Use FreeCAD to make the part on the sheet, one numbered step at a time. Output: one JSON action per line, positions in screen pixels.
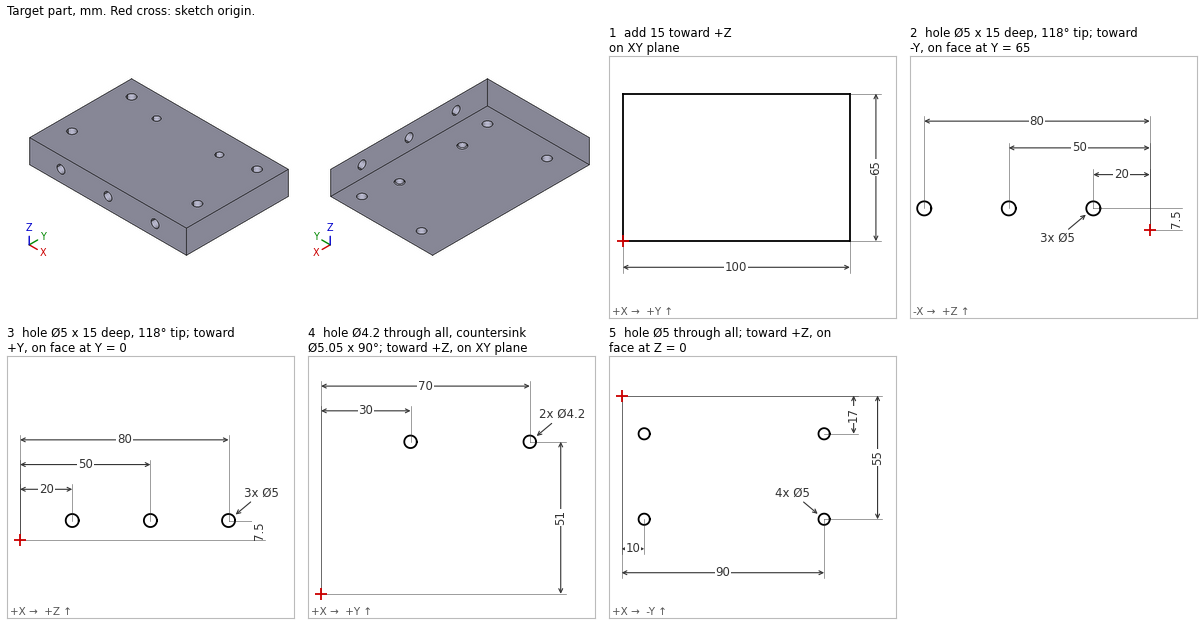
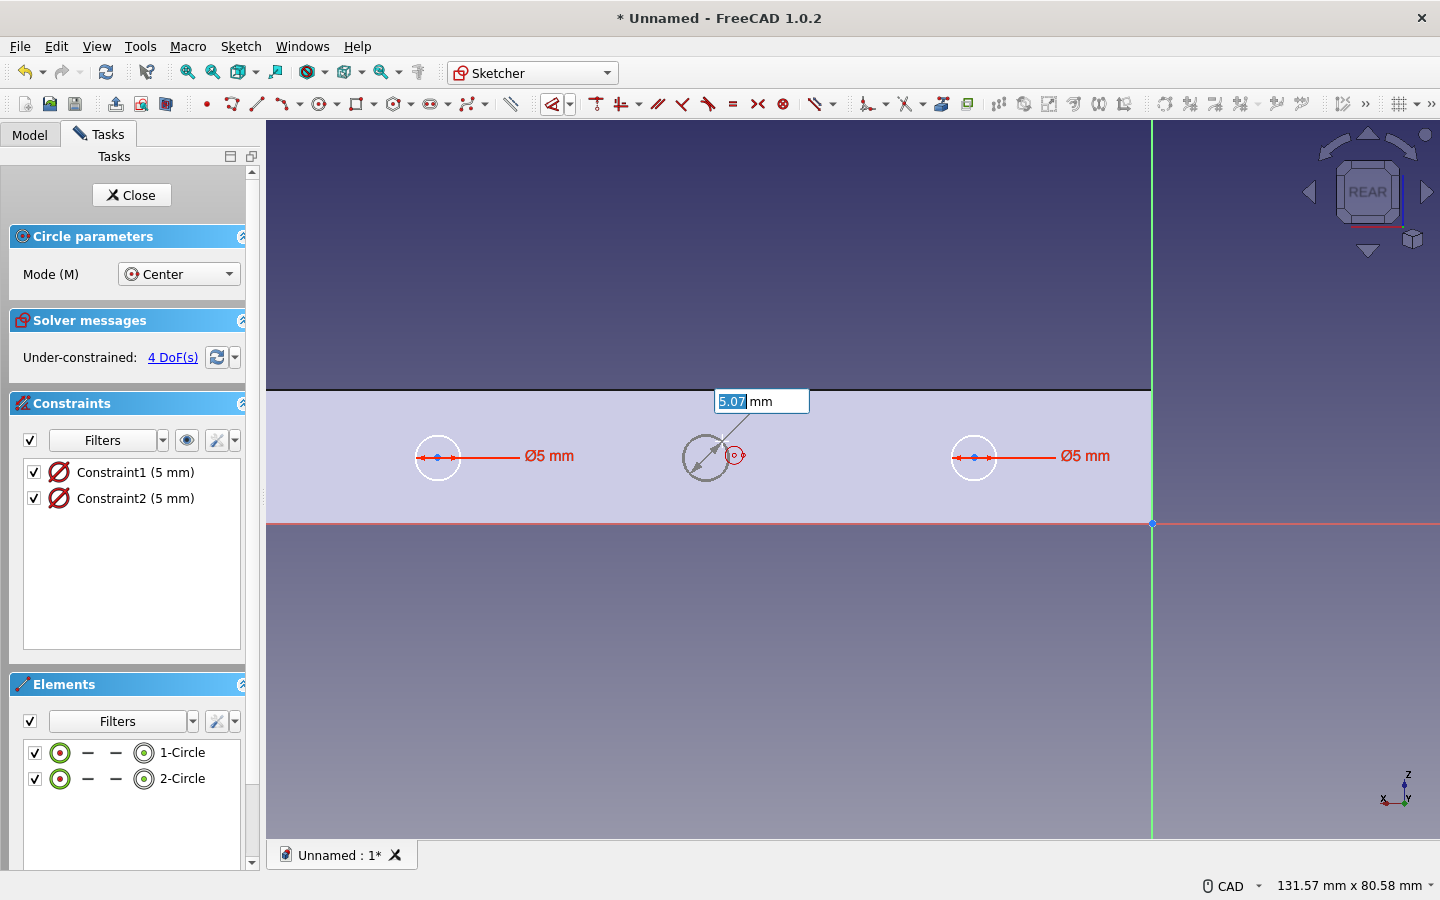
{"action": "type", "text": "5"}
{"action": "key", "text": "Return"}
{"action": "key", "text": "Escape"}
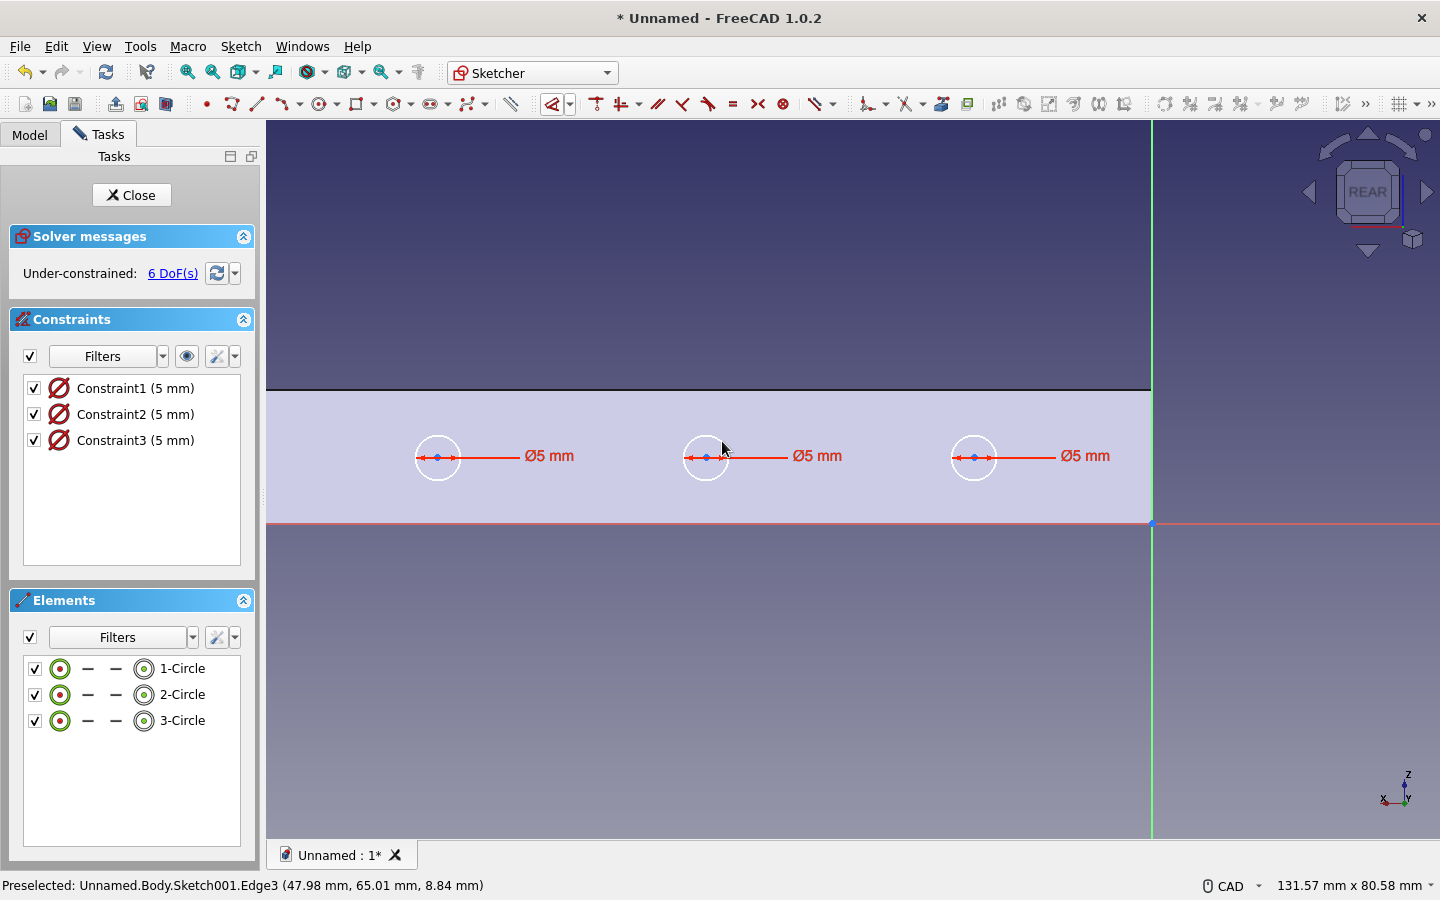
{"action": "left_click", "coordinate": [974, 458]}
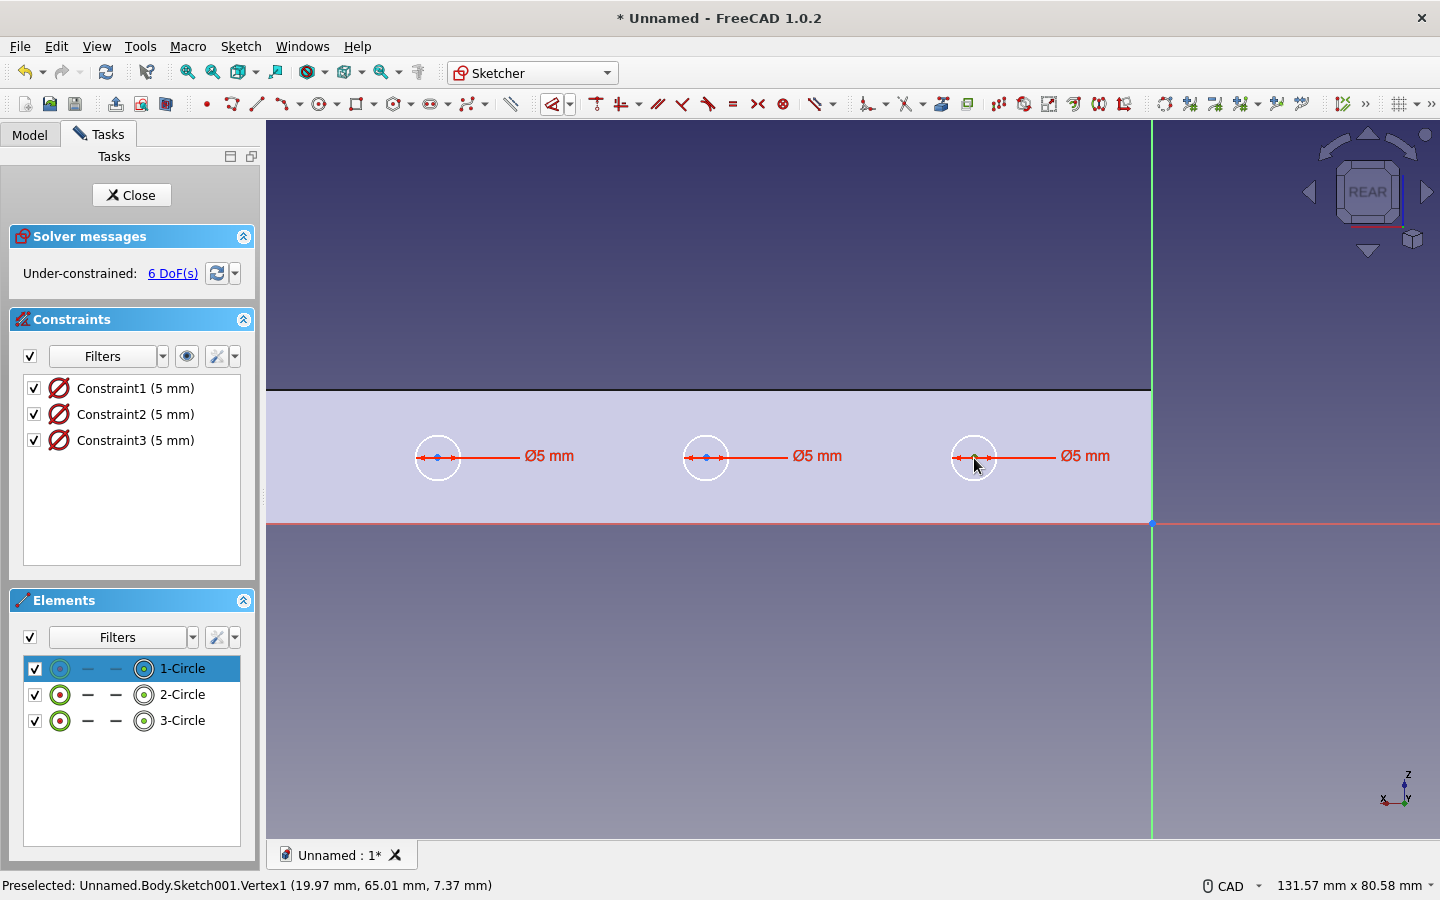
{"action": "left_click", "coordinate": [438, 458]}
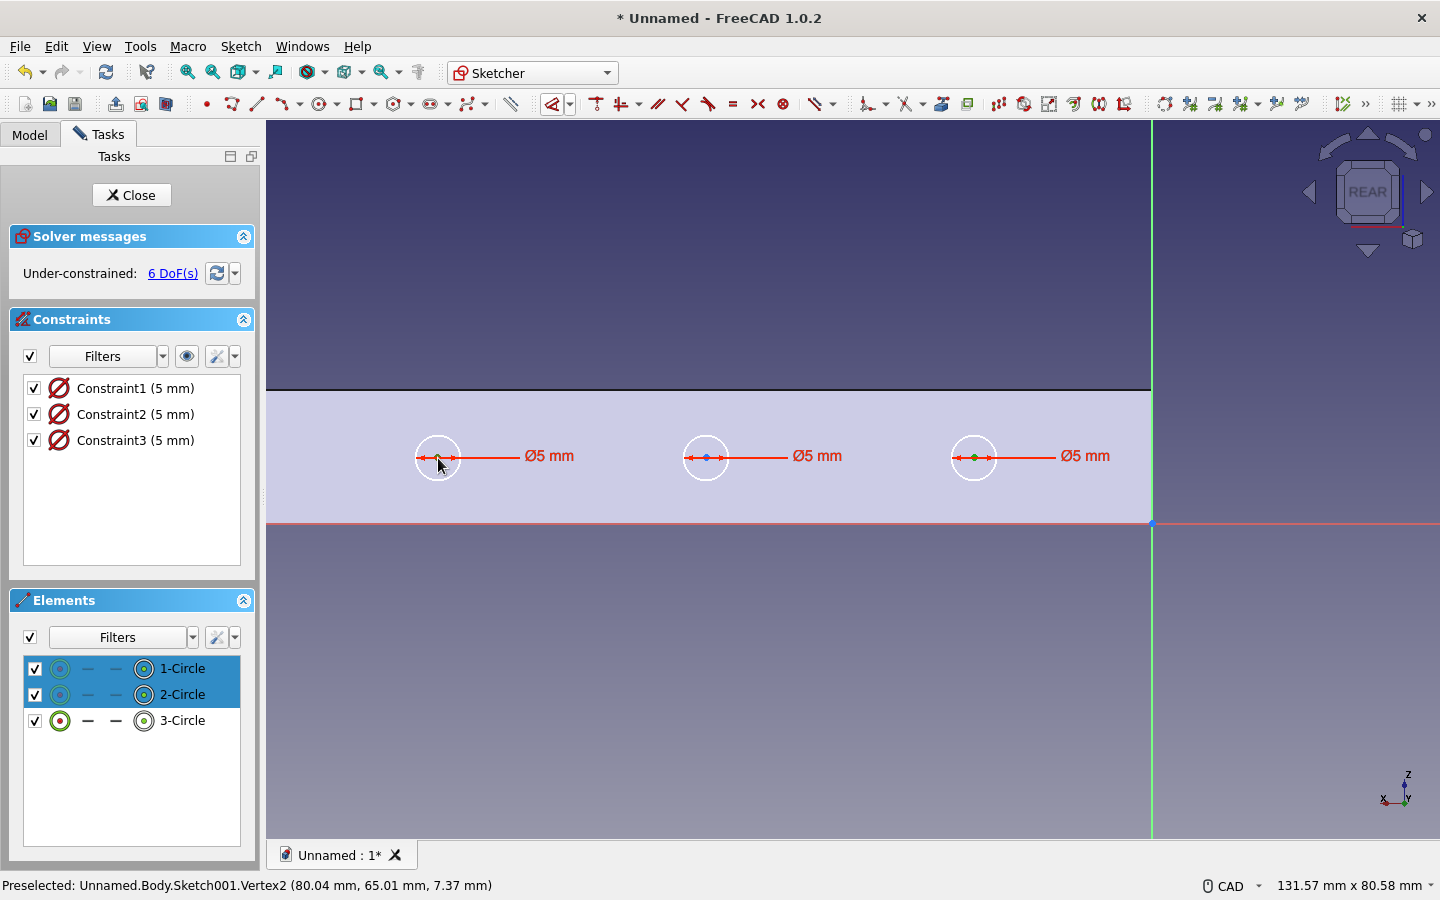
{"action": "key", "text": "h"}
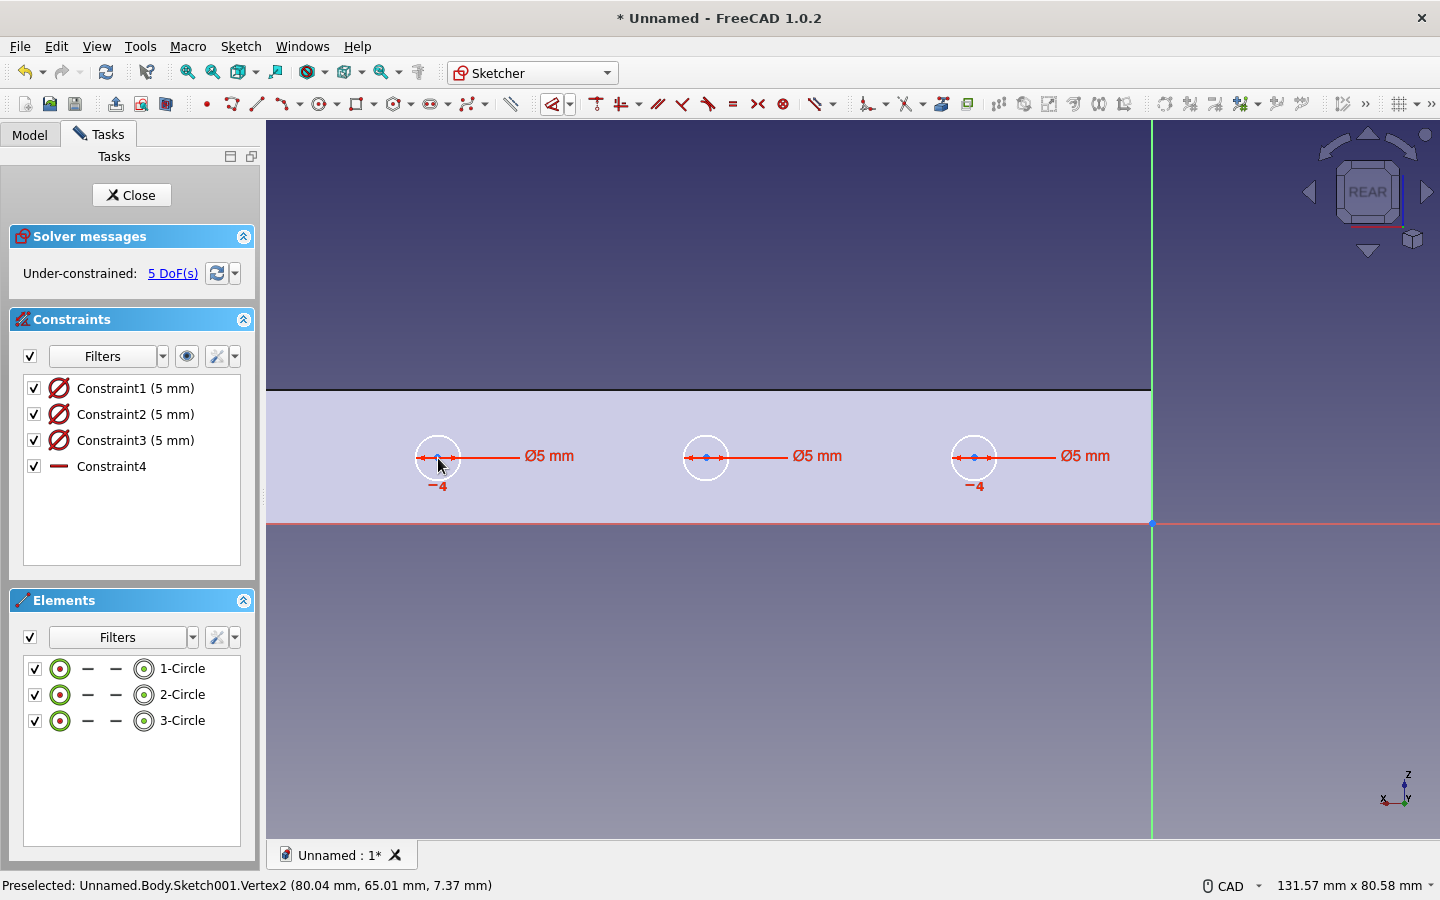
{"action": "left_click", "coordinate": [974, 458]}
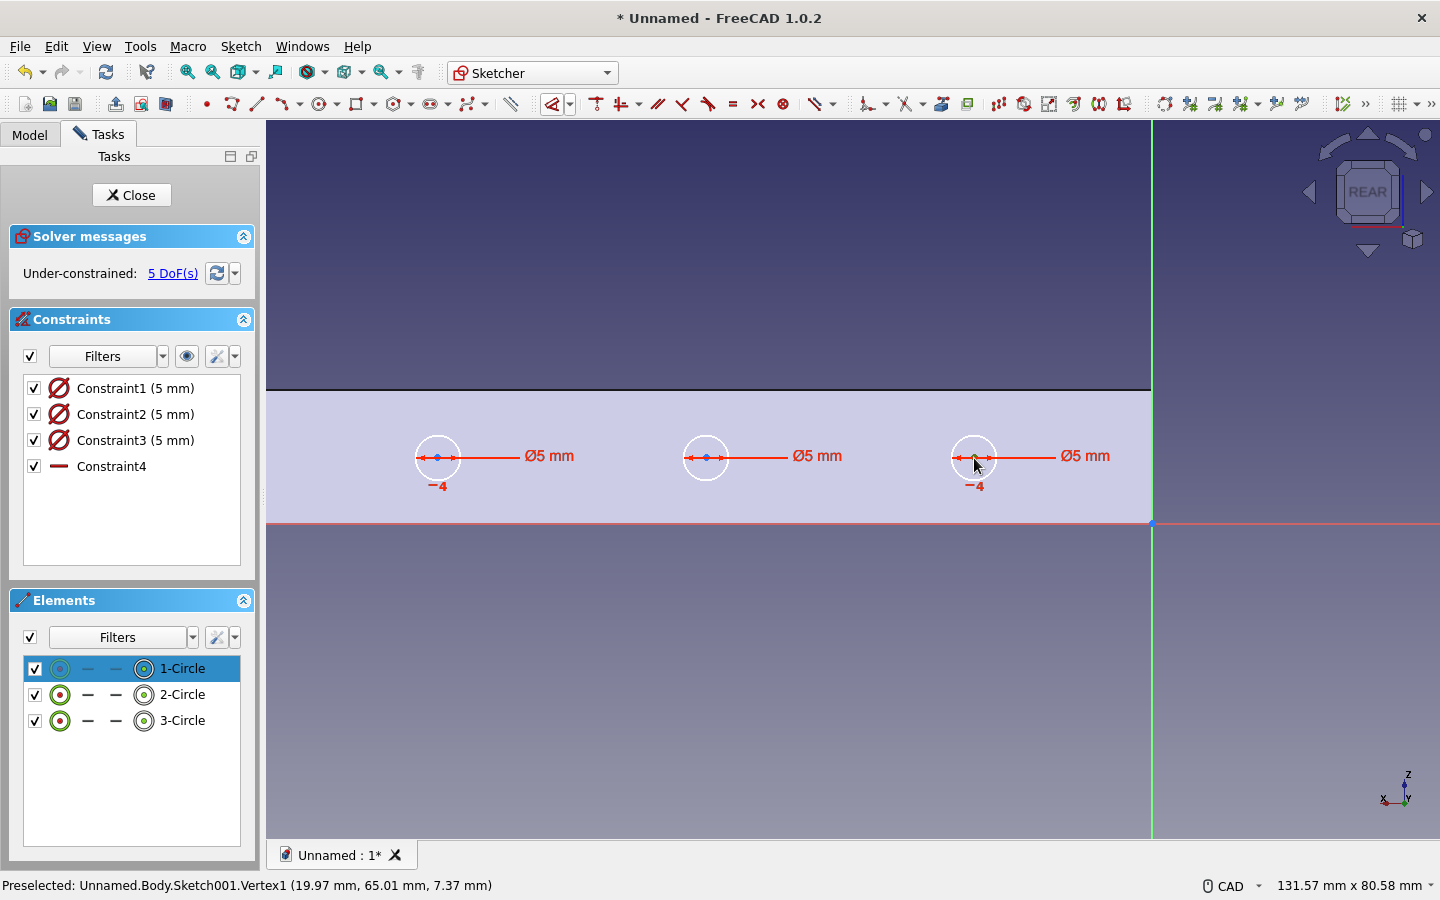
{"action": "left_click", "coordinate": [706, 458]}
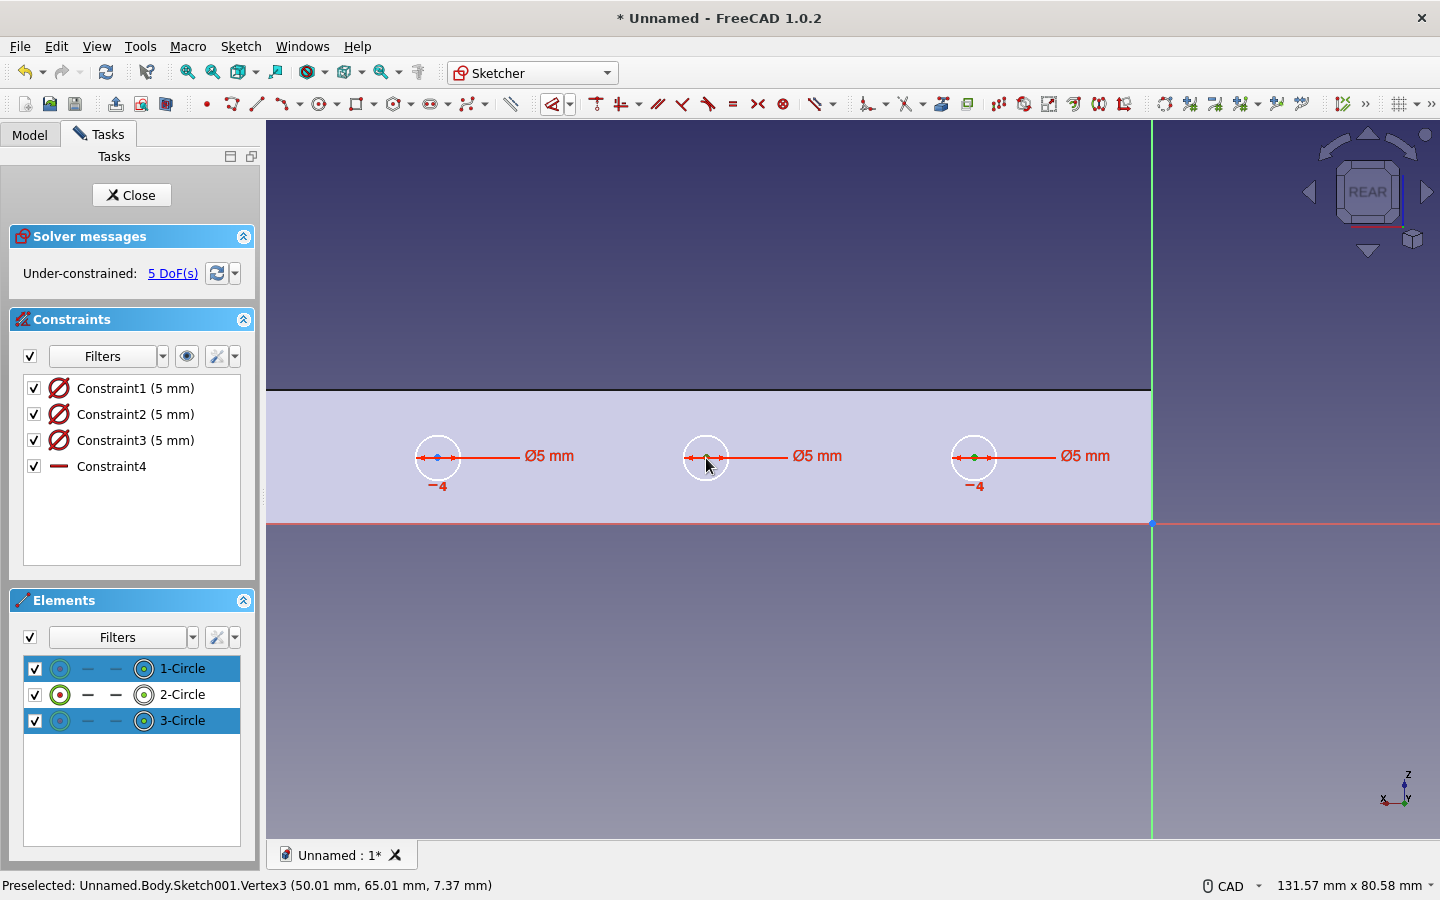
{"action": "left_click", "coordinate": [638, 104]}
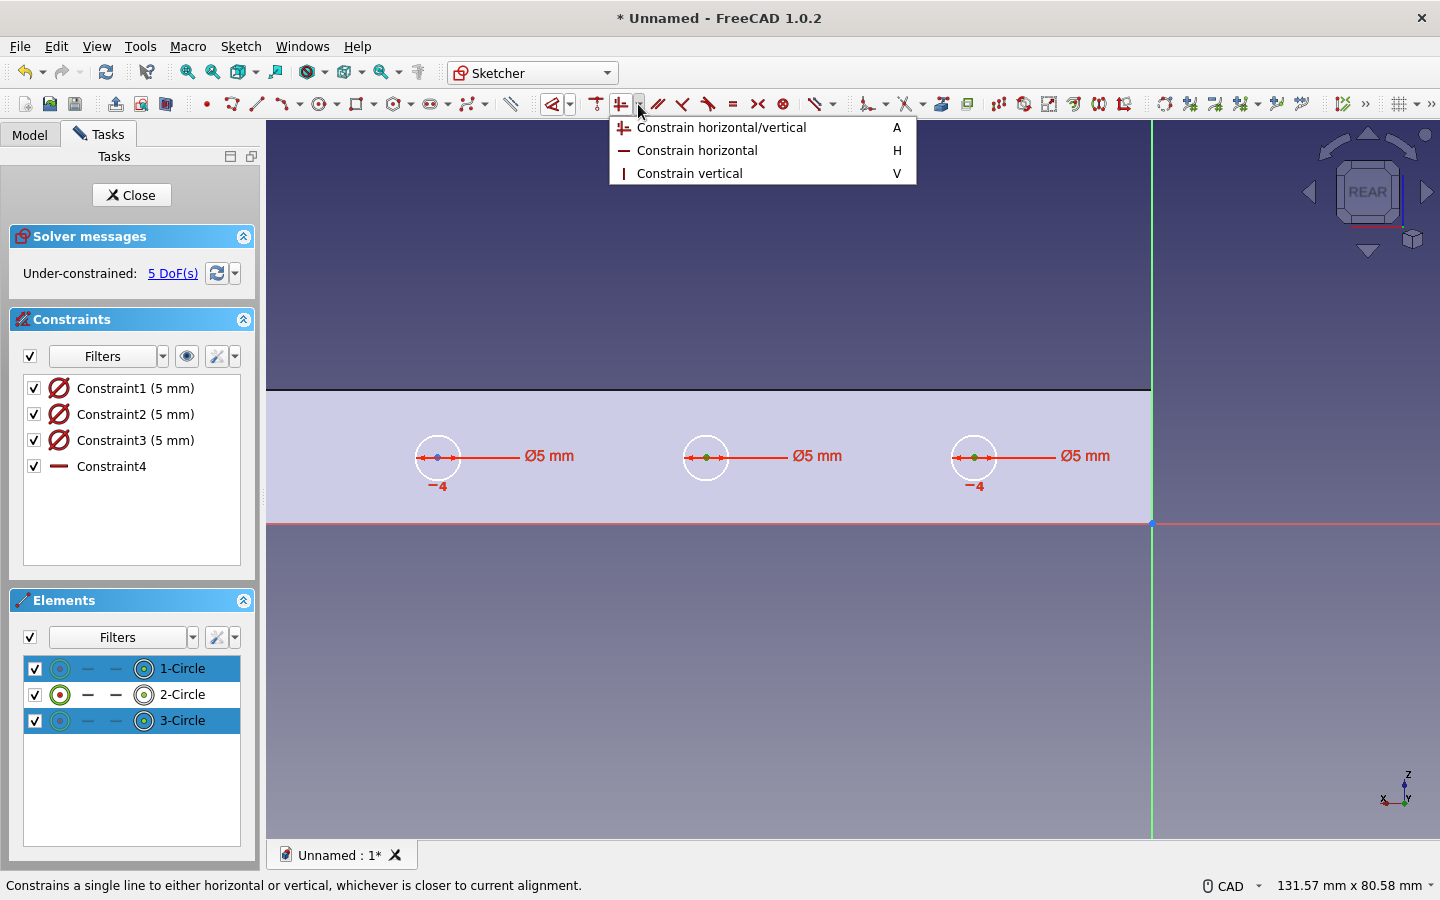
{"action": "left_click", "coordinate": [763, 150]}